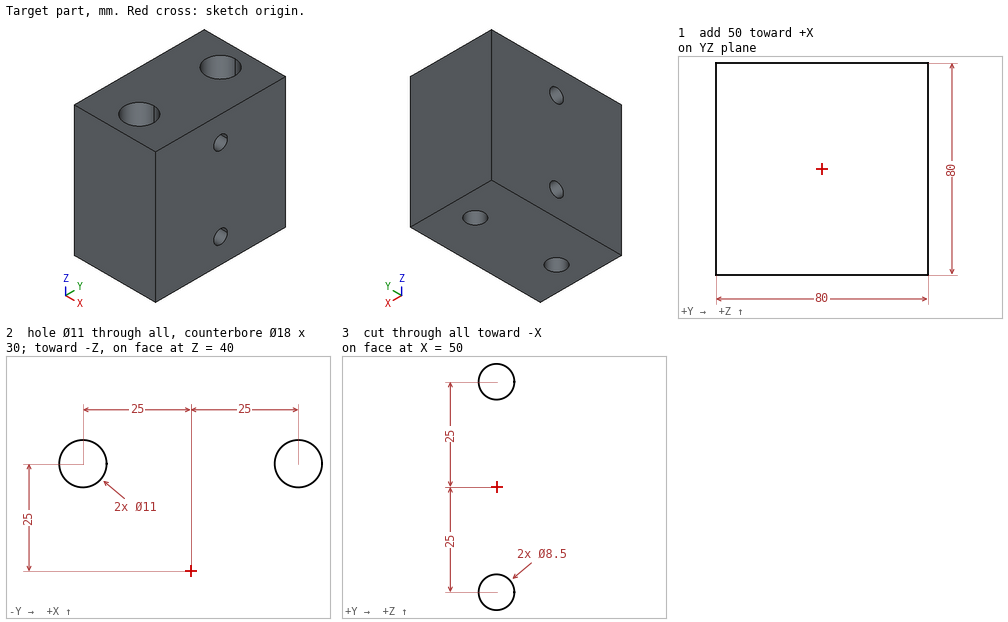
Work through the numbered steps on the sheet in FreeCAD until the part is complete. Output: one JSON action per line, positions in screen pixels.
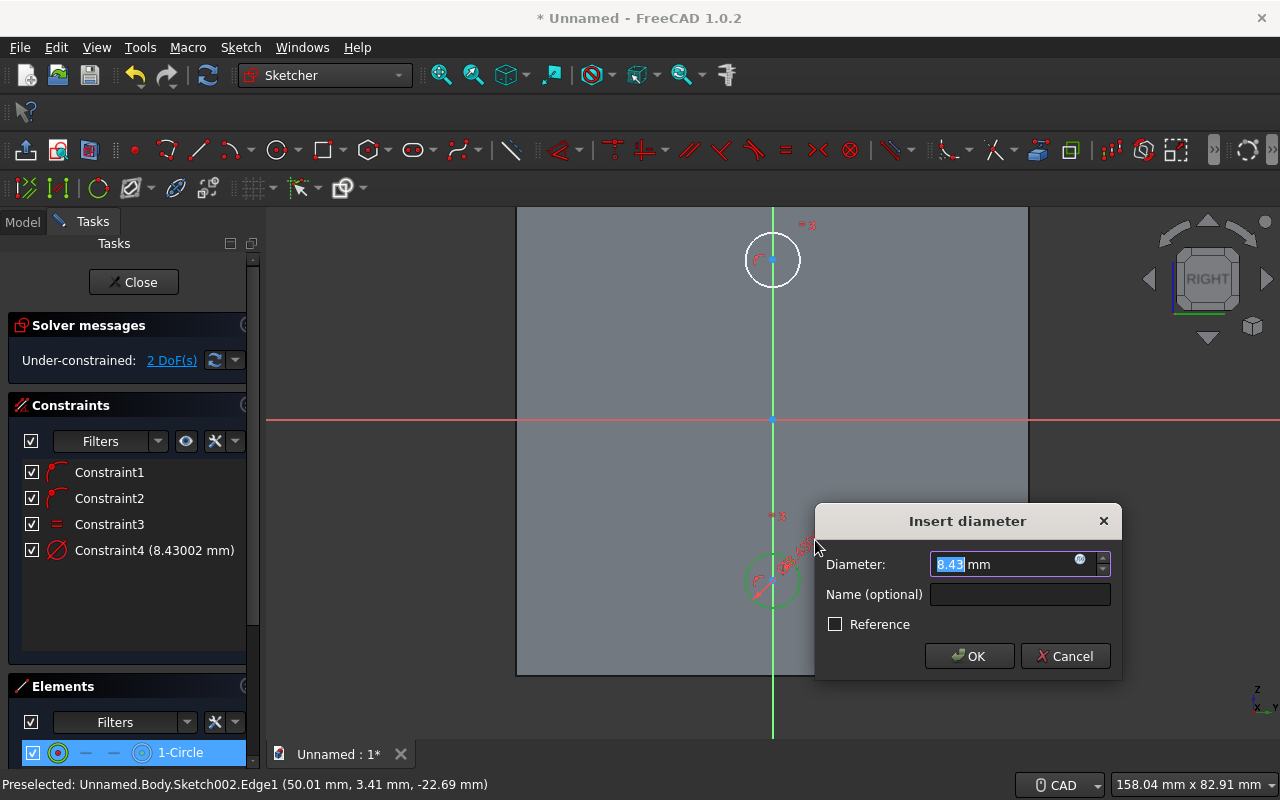
{"action": "type", "text": "8.5"}
{"action": "key", "text": "Return"}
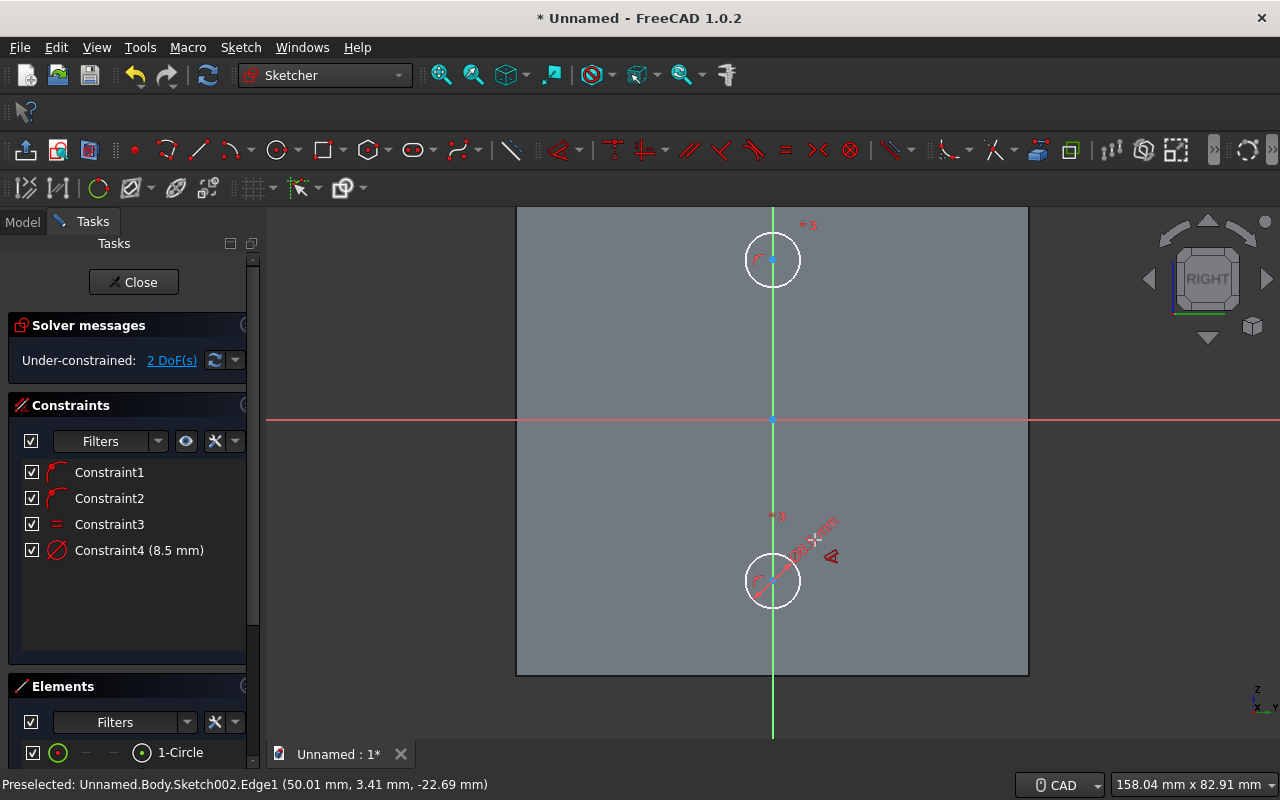
{"action": "left_click", "coordinate": [773, 581]}
{"action": "left_click", "coordinate": [807, 500]}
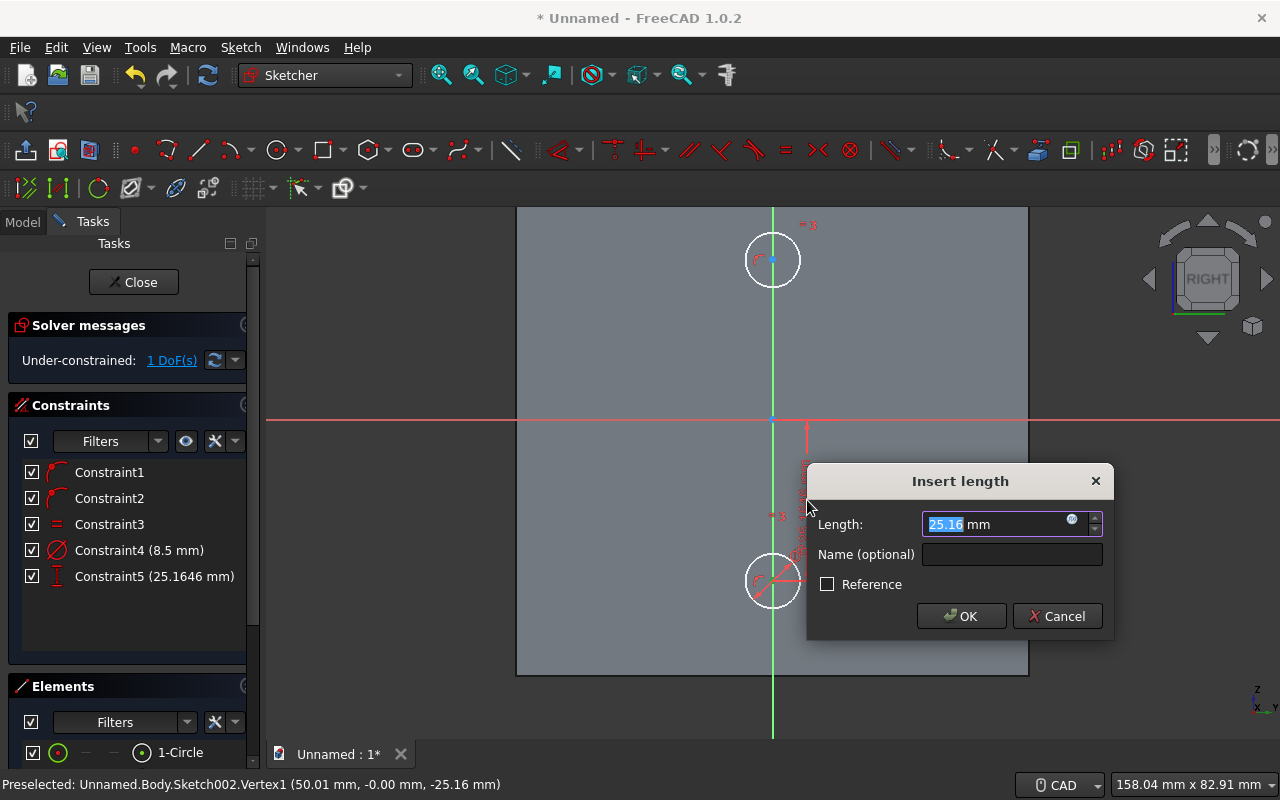
{"action": "type", "text": "25"}
{"action": "key", "text": "Return"}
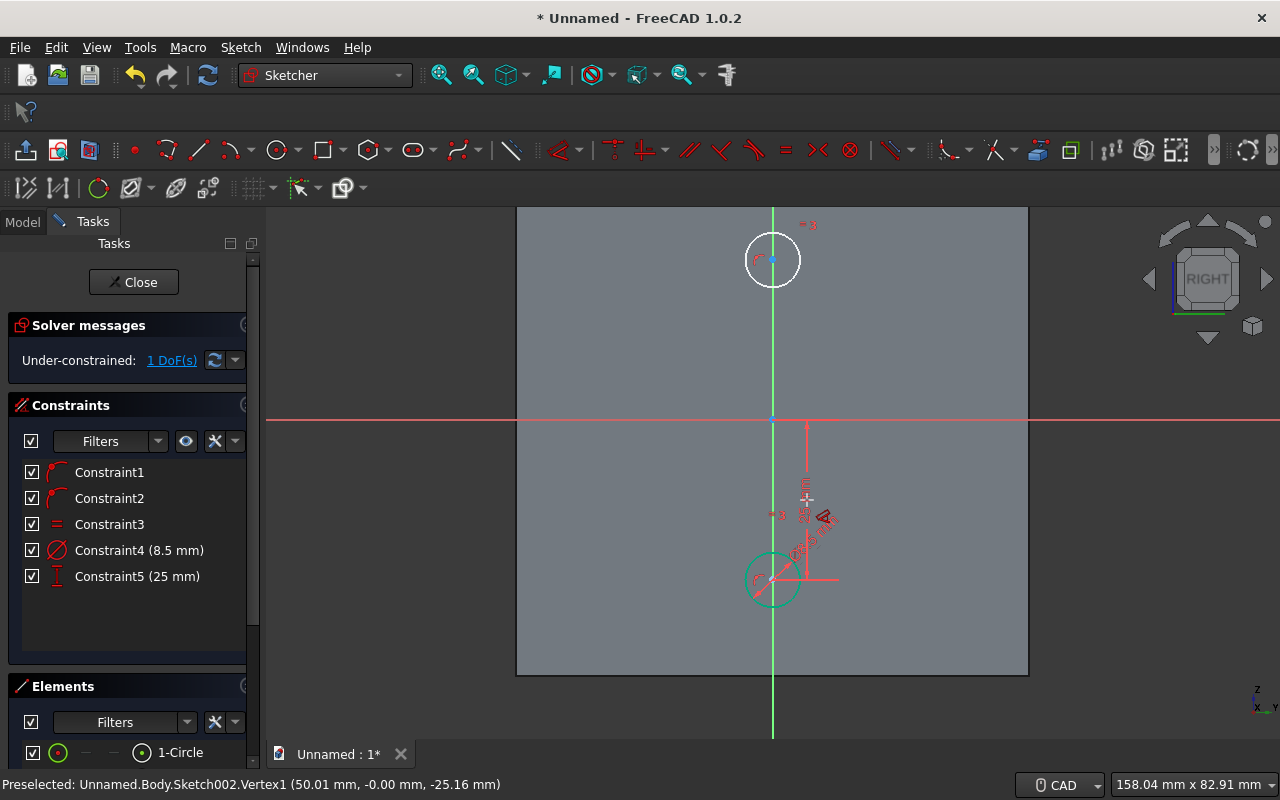
{"action": "left_click", "coordinate": [773, 260]}
{"action": "left_click", "coordinate": [807, 340]}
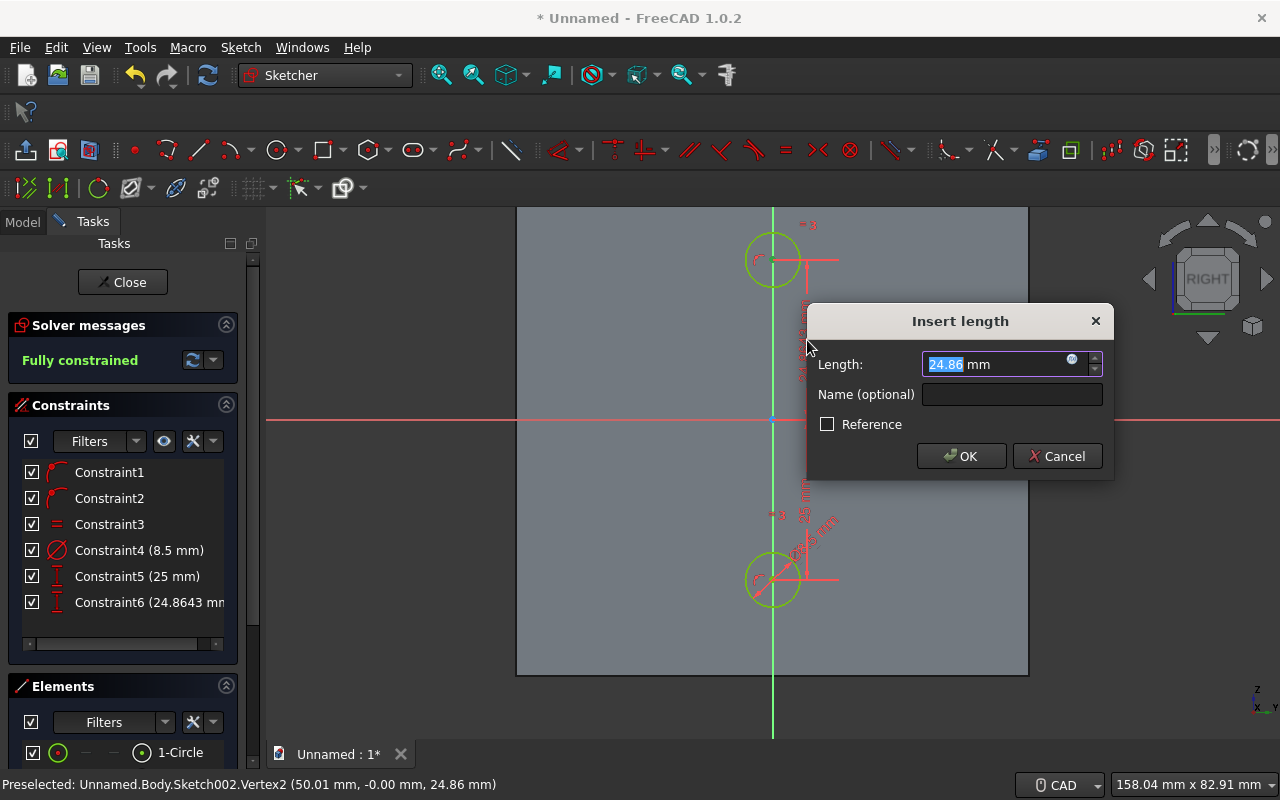
{"action": "type", "text": "25"}
{"action": "key", "text": "Return"}
{"action": "key", "text": "Escape"}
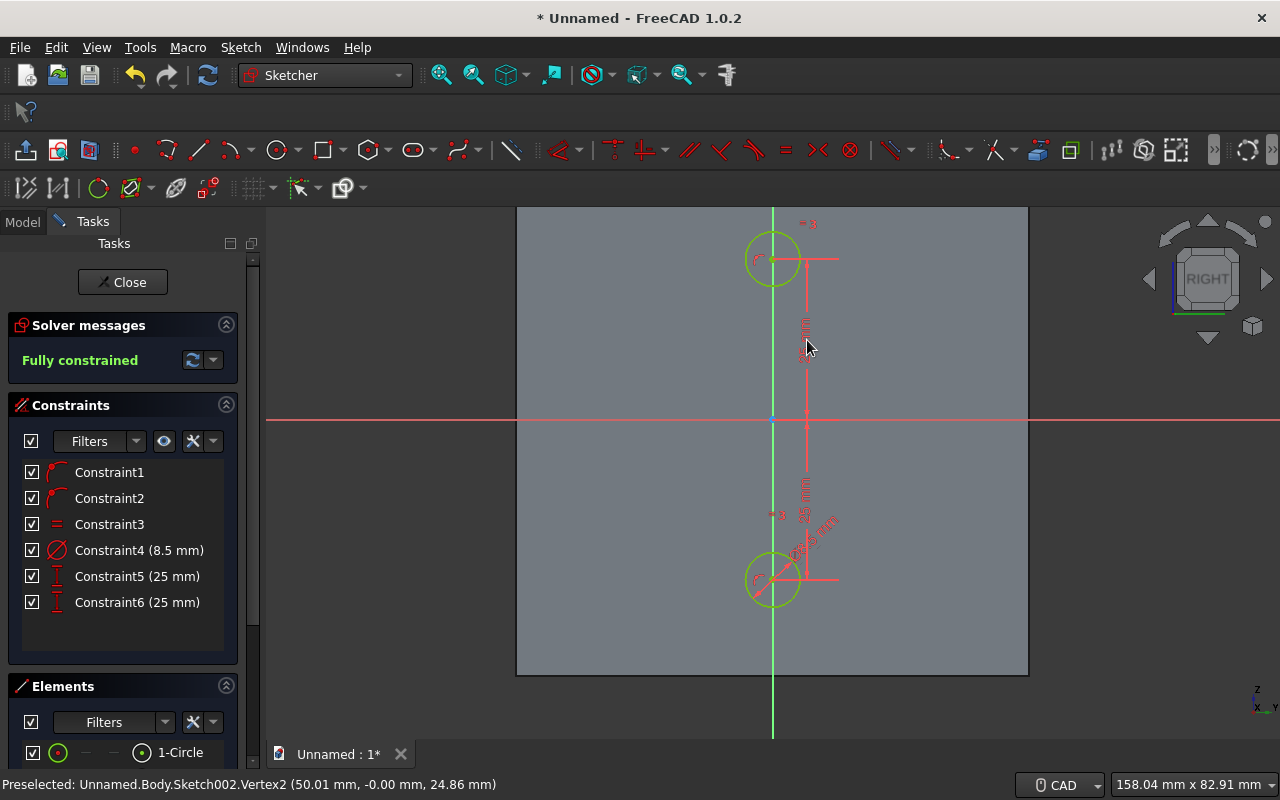
{"action": "left_click", "coordinate": [123, 282]}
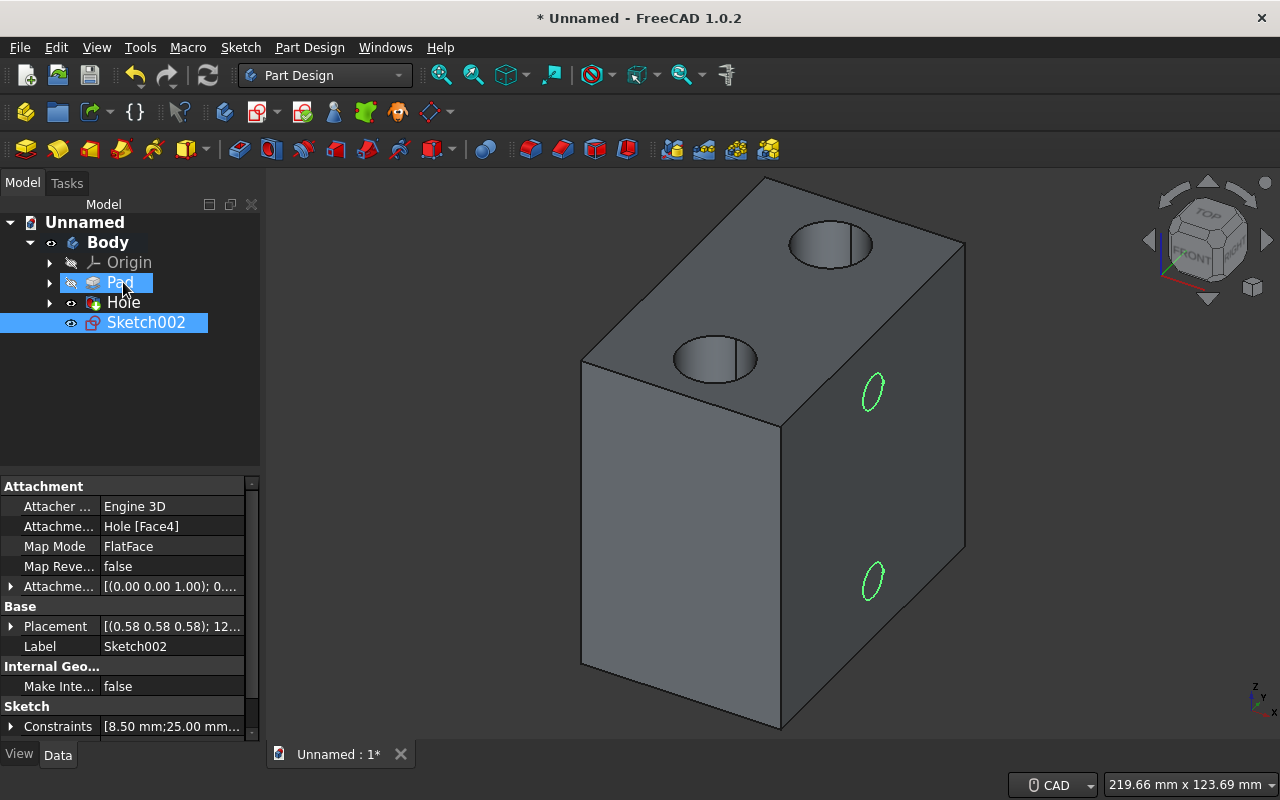
{"action": "left_click", "coordinate": [240, 150]}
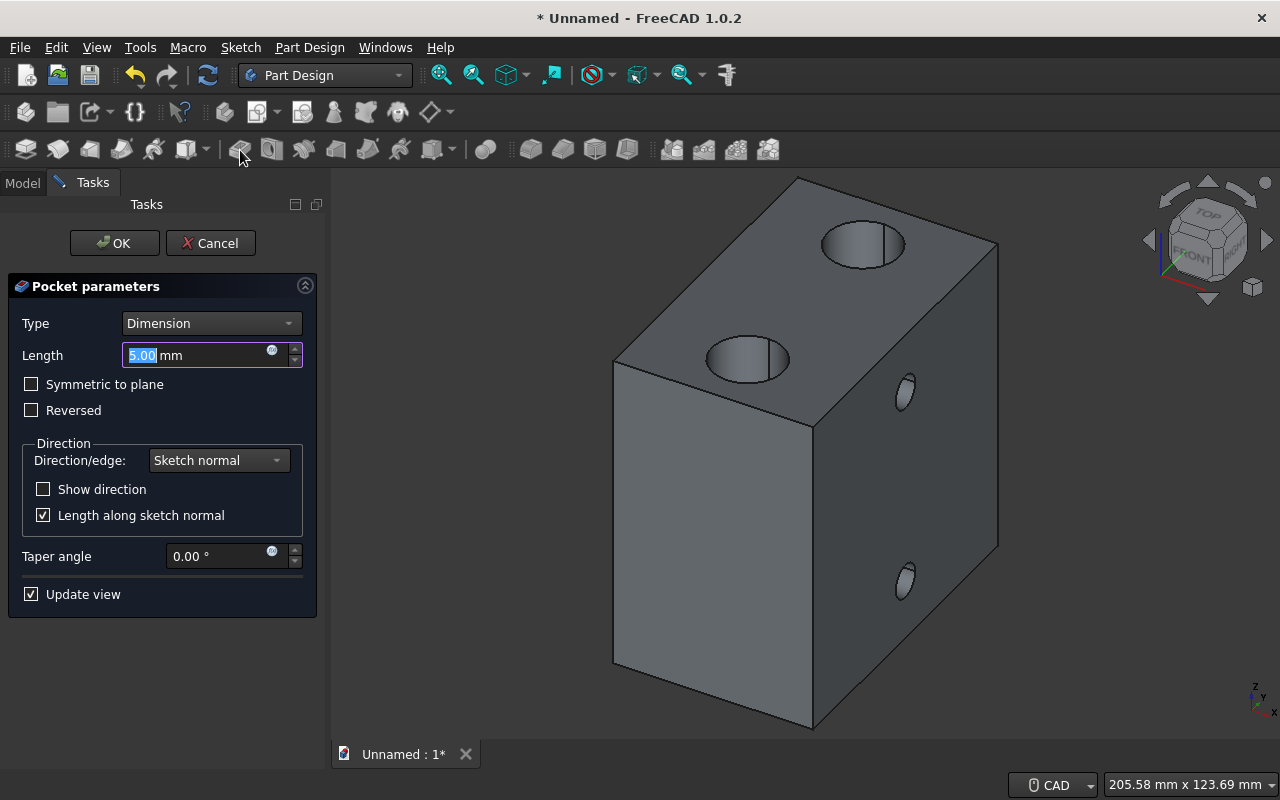
{"action": "left_click", "coordinate": [212, 324]}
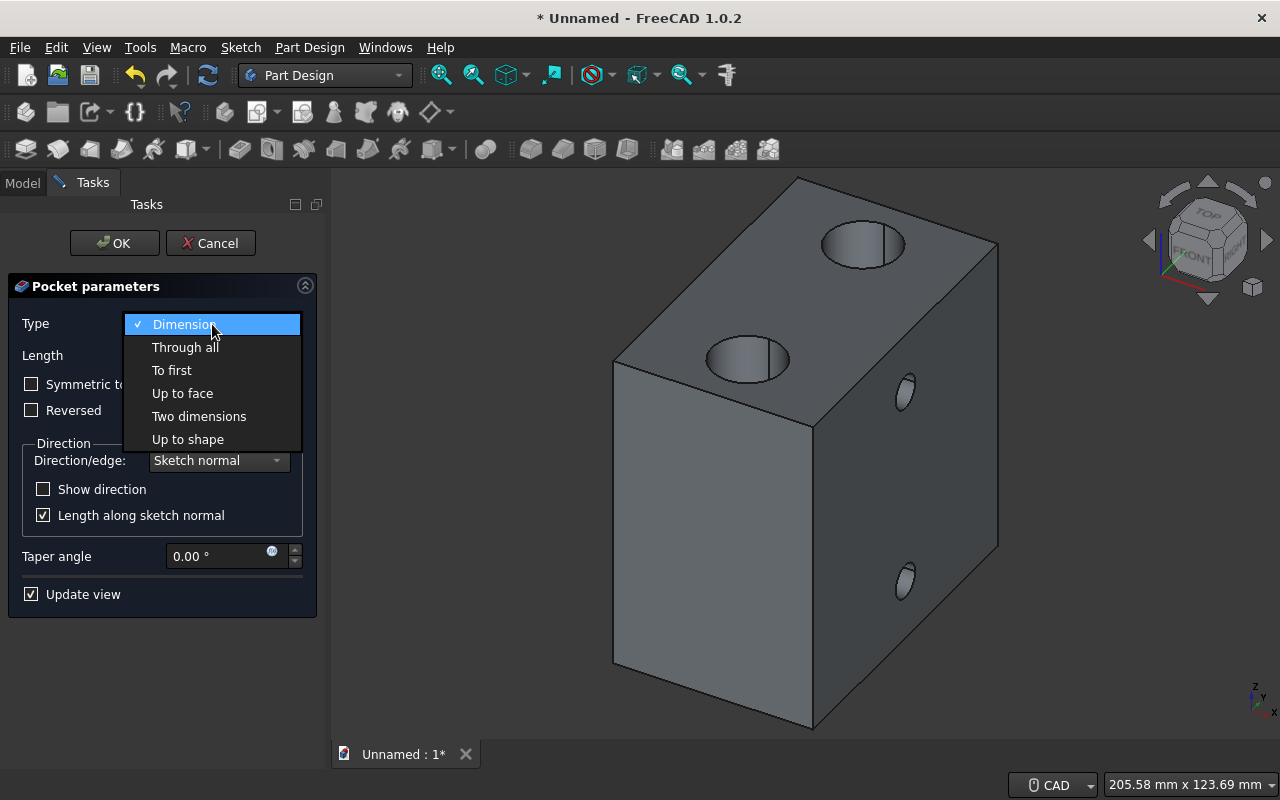
{"action": "left_click", "coordinate": [212, 348]}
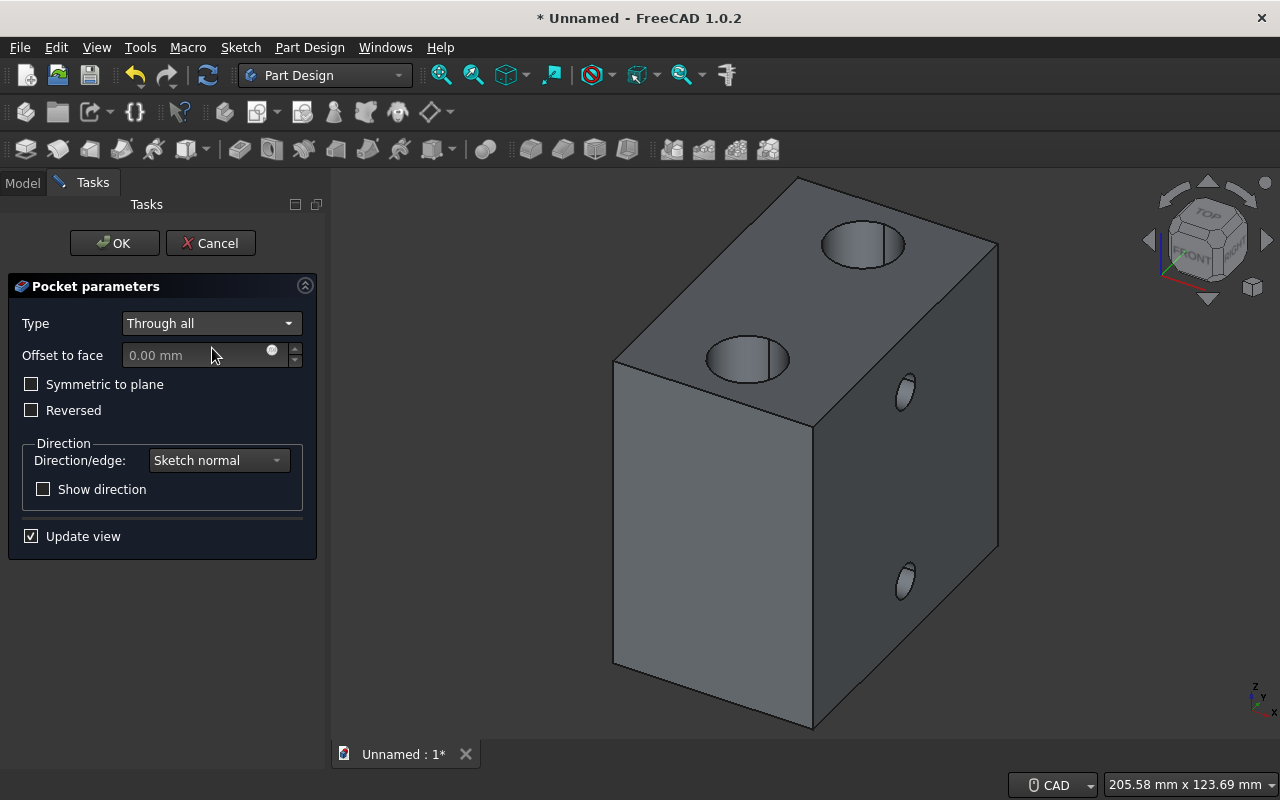
{"action": "left_click", "coordinate": [115, 243]}